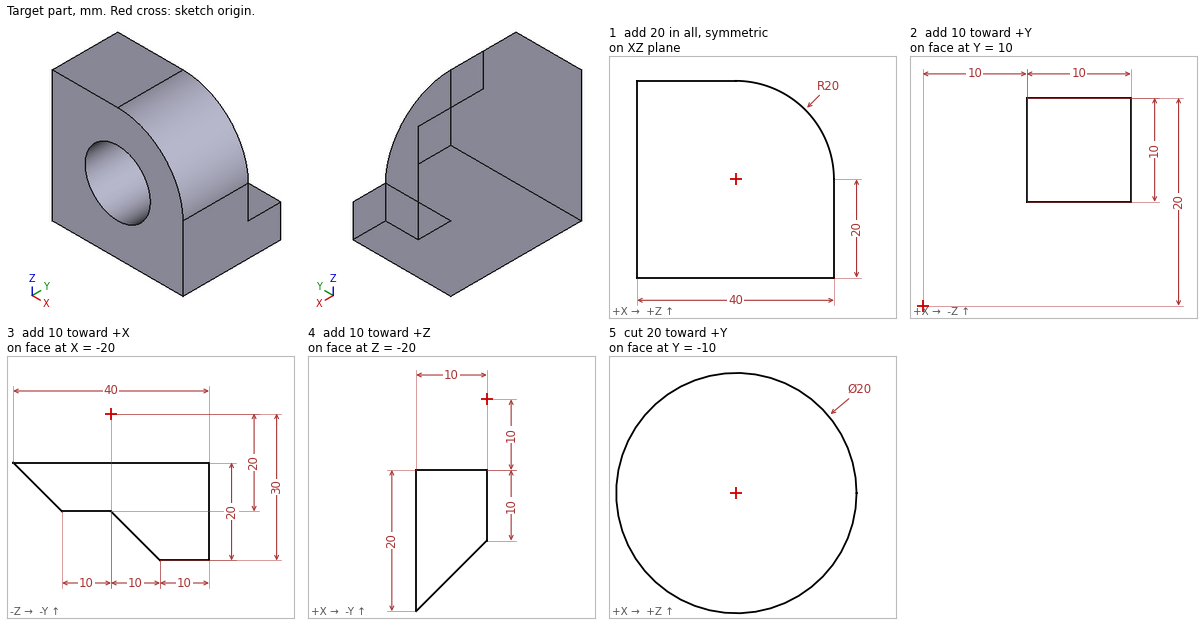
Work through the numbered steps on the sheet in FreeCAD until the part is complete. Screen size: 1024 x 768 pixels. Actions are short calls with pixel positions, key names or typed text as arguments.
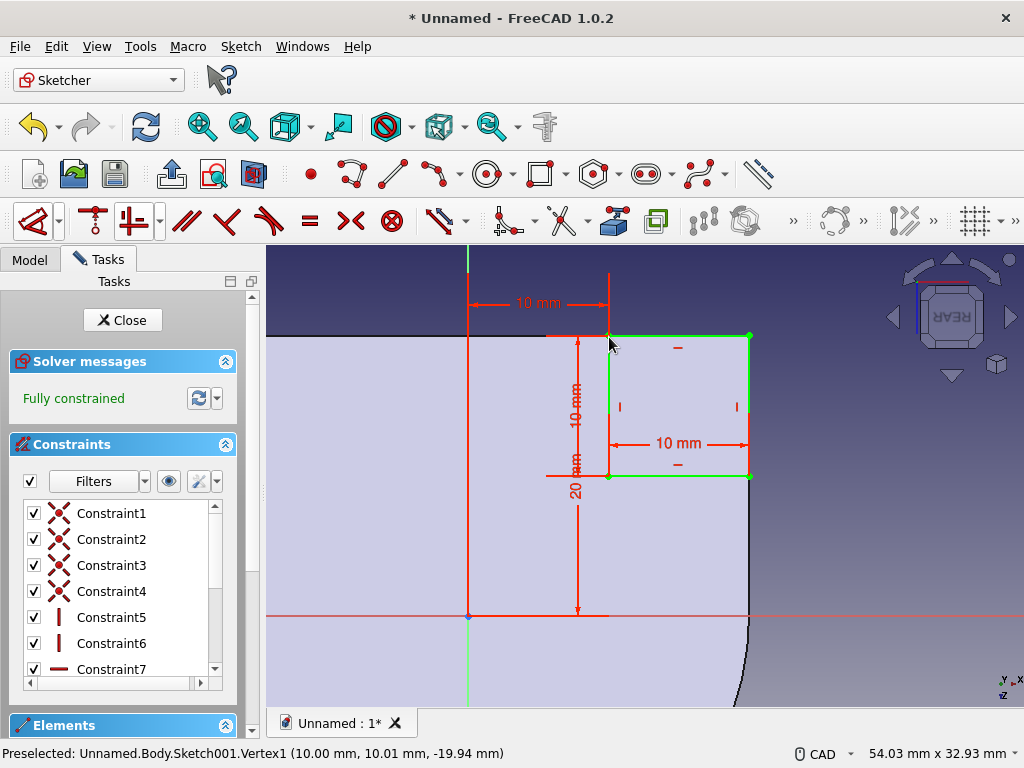
click(123, 320)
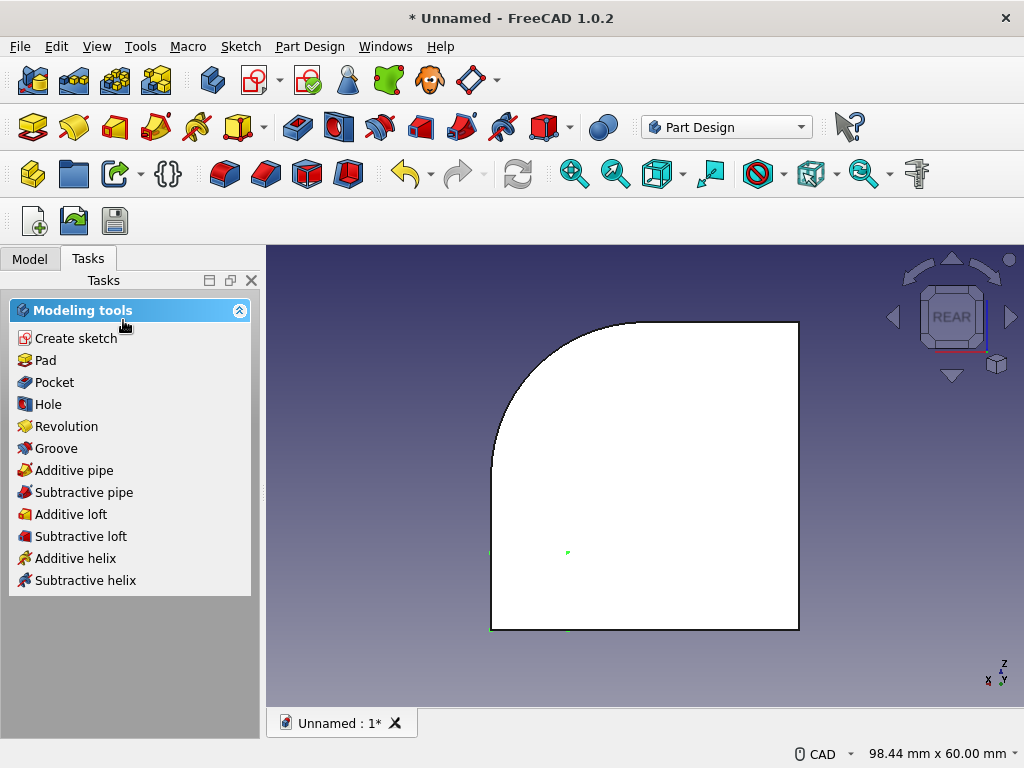
click(33, 128)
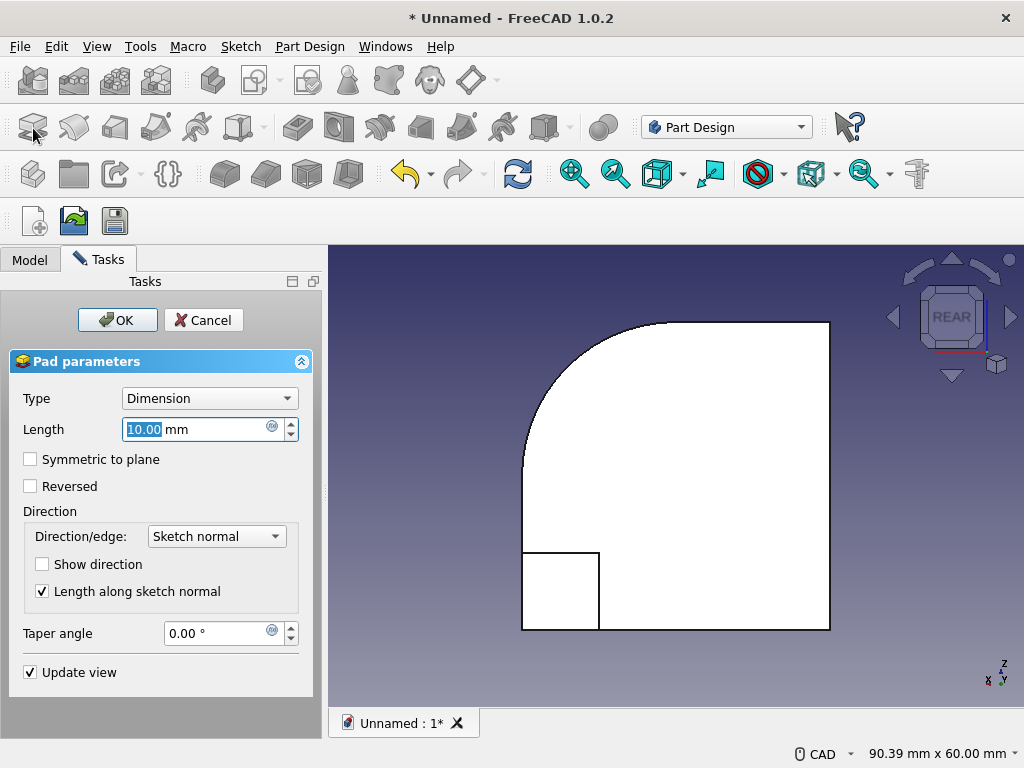
text(10)
key(Tab)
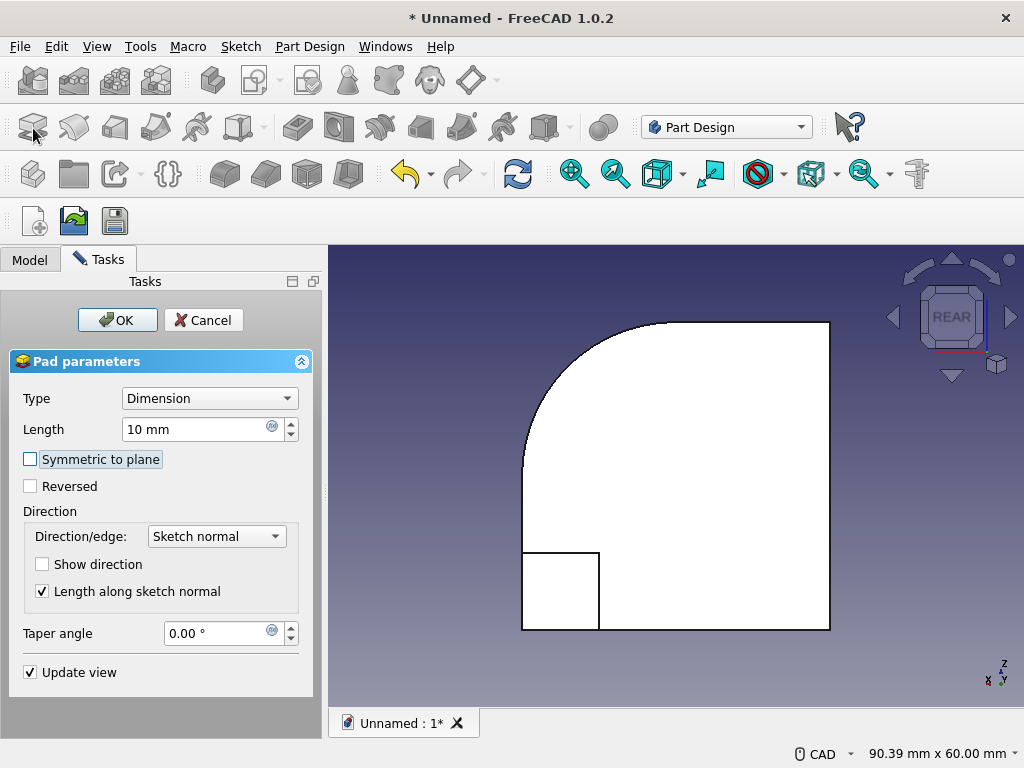
click(118, 320)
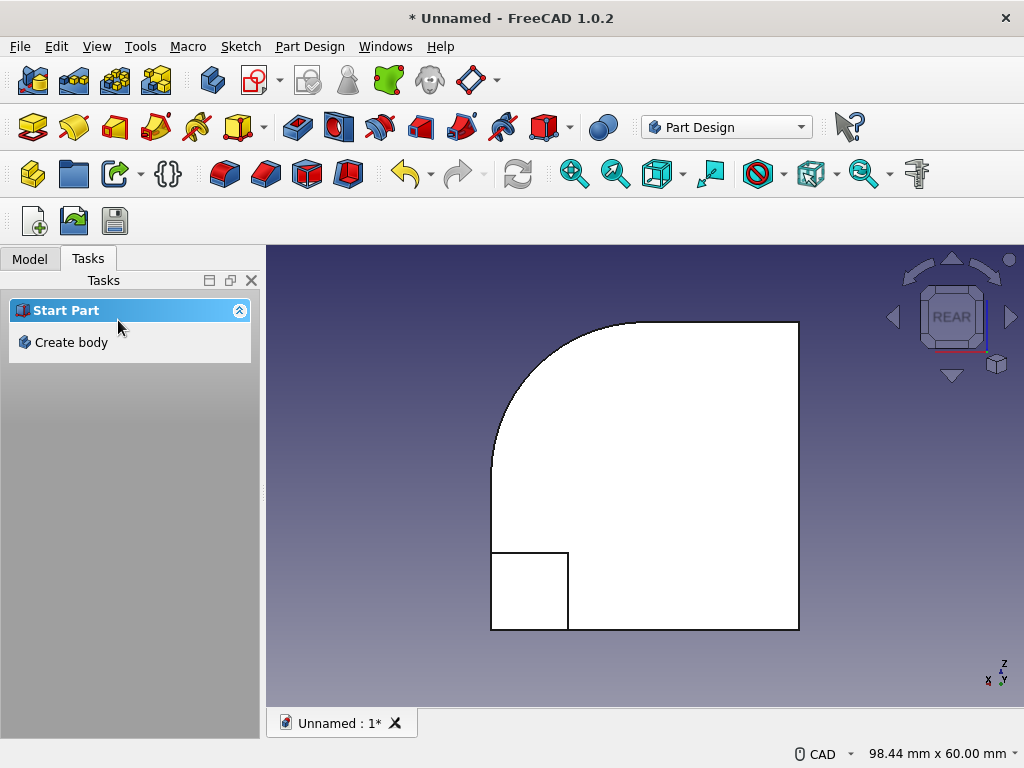
key(6)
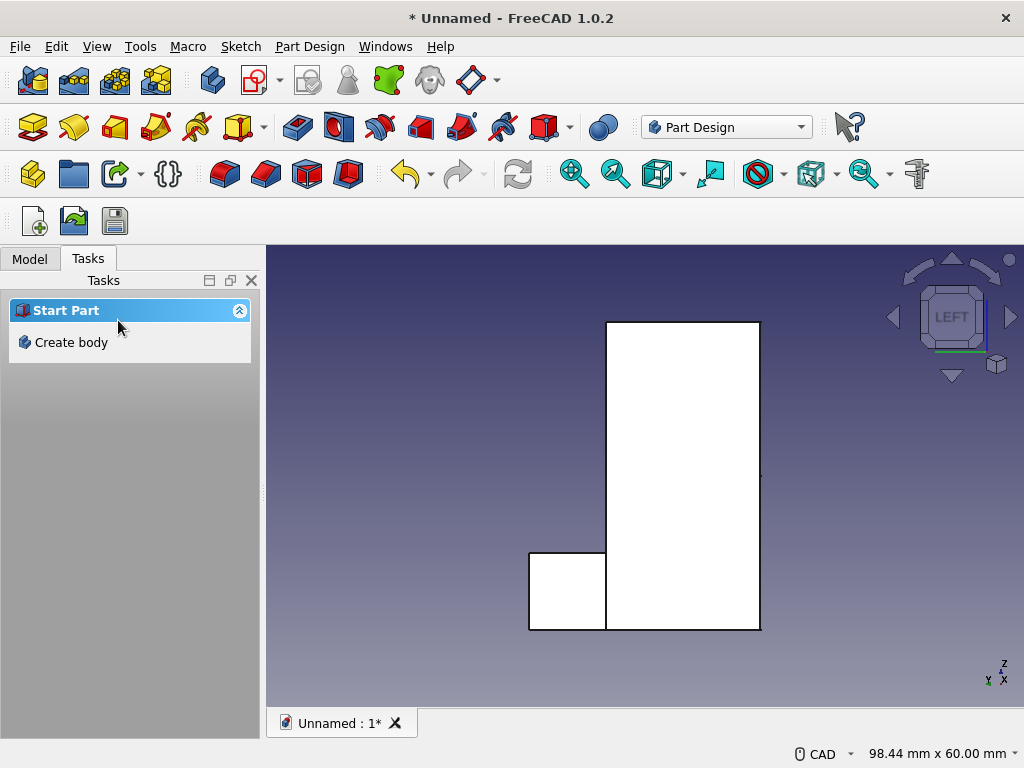
click(683, 431)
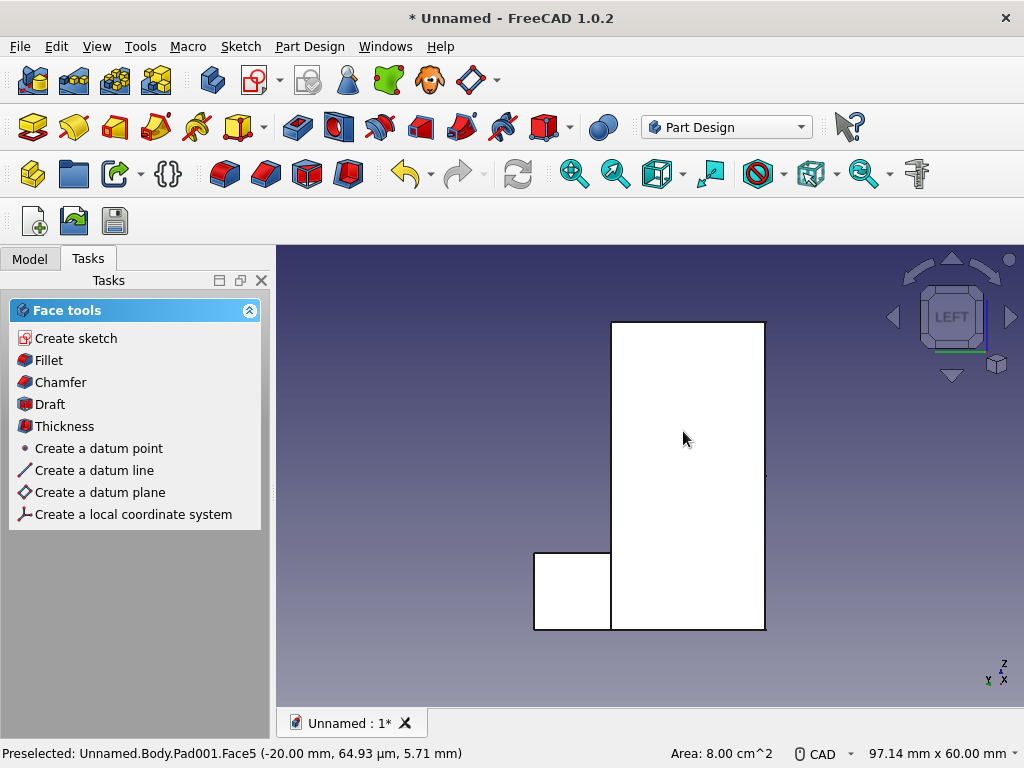
click(254, 80)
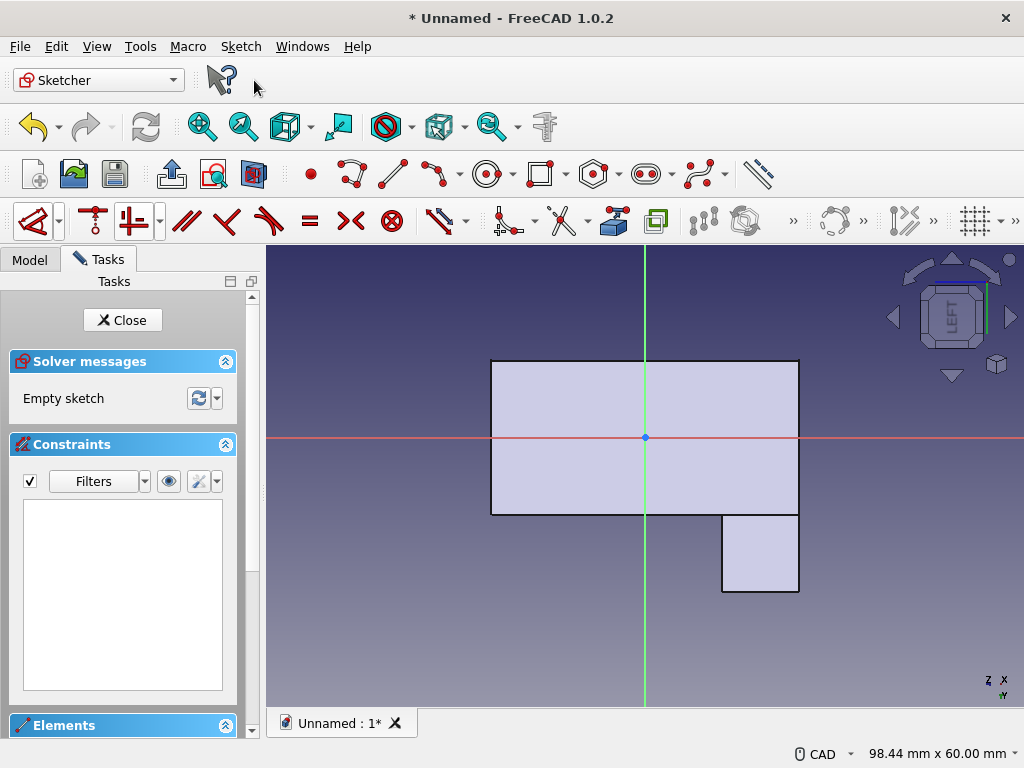
scroll(294, 273, down, 1)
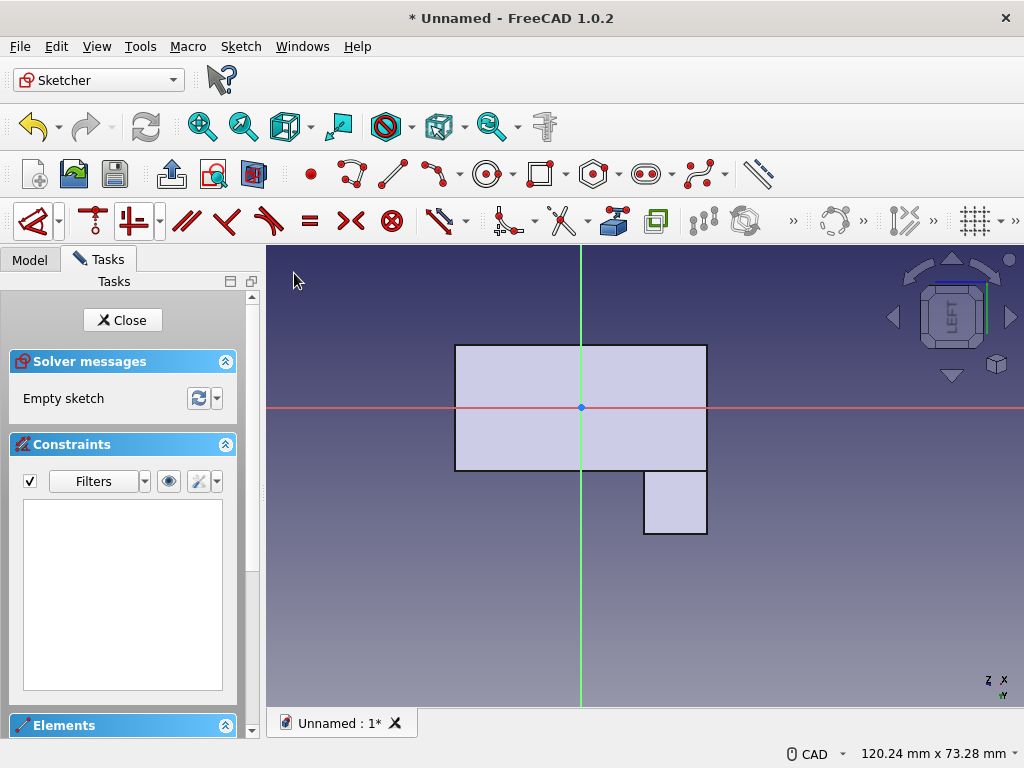
scroll(591, 556, up, 2)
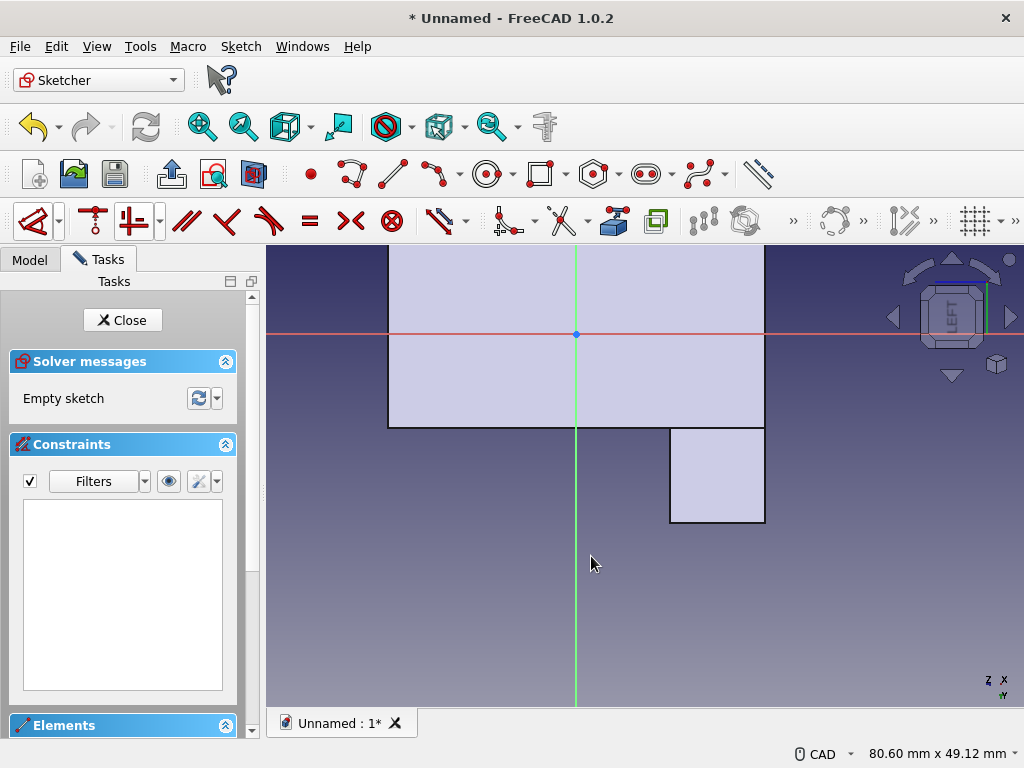
click(352, 174)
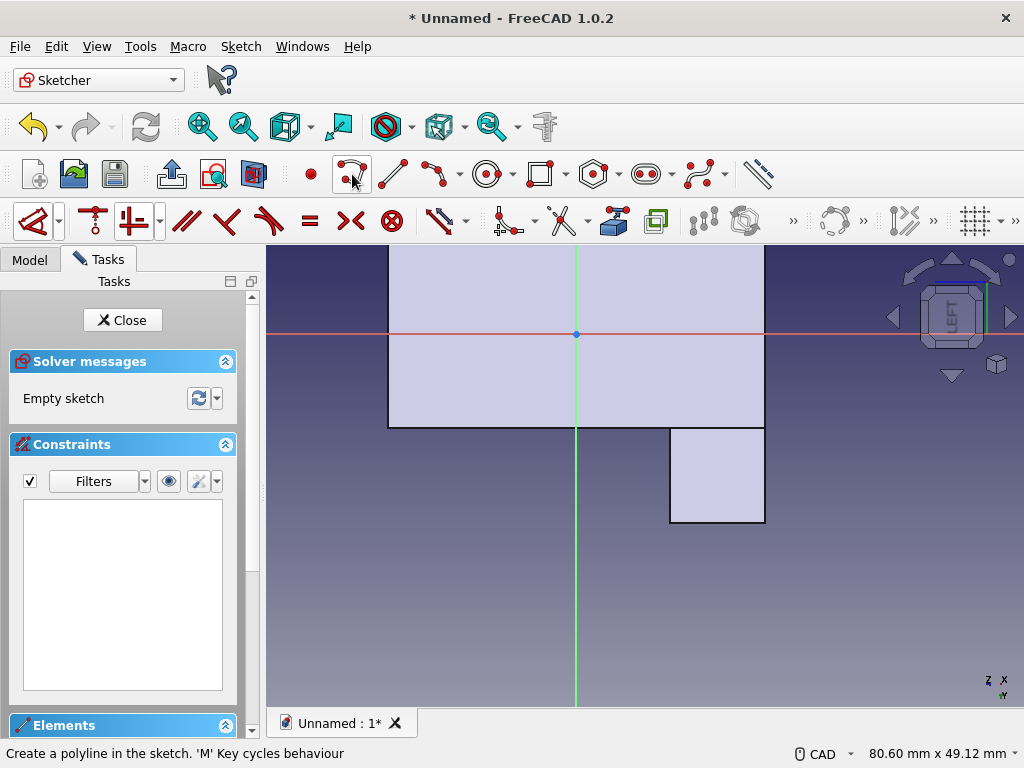
click(576, 523)
click(670, 617)
click(765, 617)
click(765, 428)
click(388, 428)
click(482, 523)
click(576, 524)
key(Escape)
key(Escape)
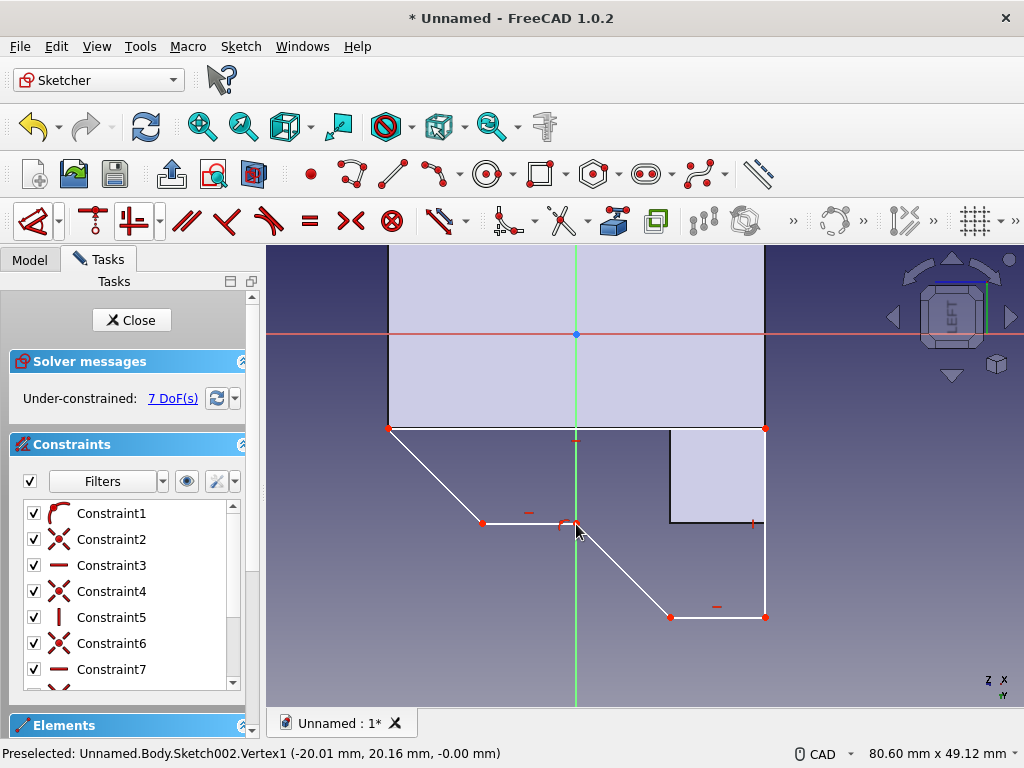
click(699, 618)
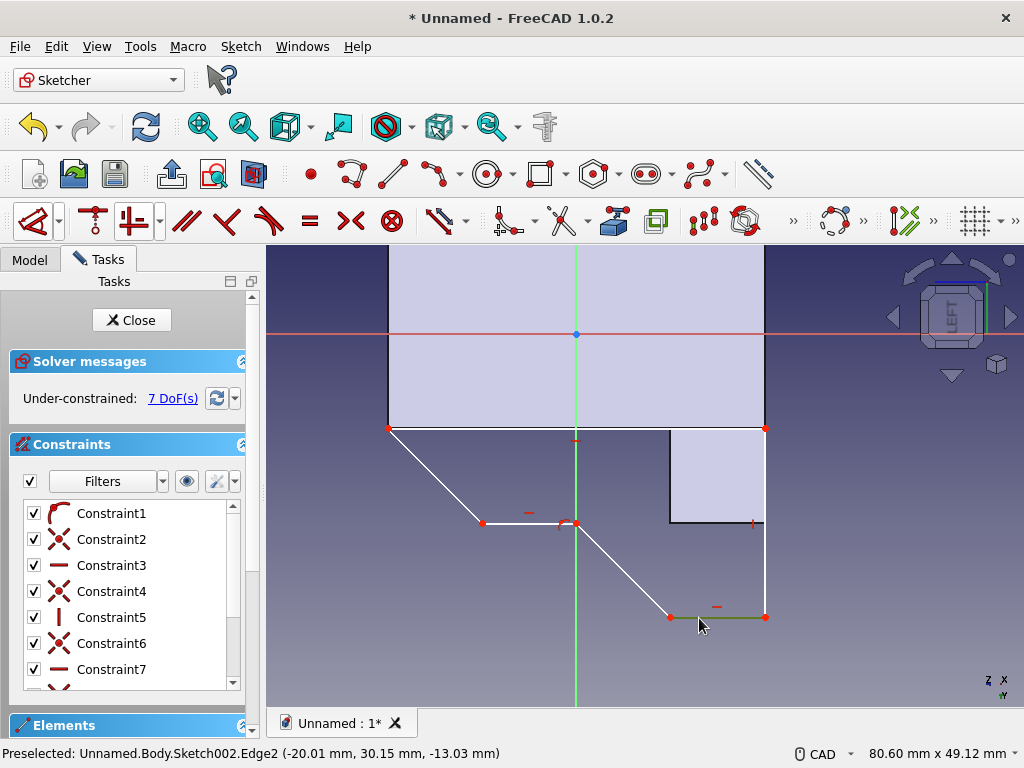
click(58, 222)